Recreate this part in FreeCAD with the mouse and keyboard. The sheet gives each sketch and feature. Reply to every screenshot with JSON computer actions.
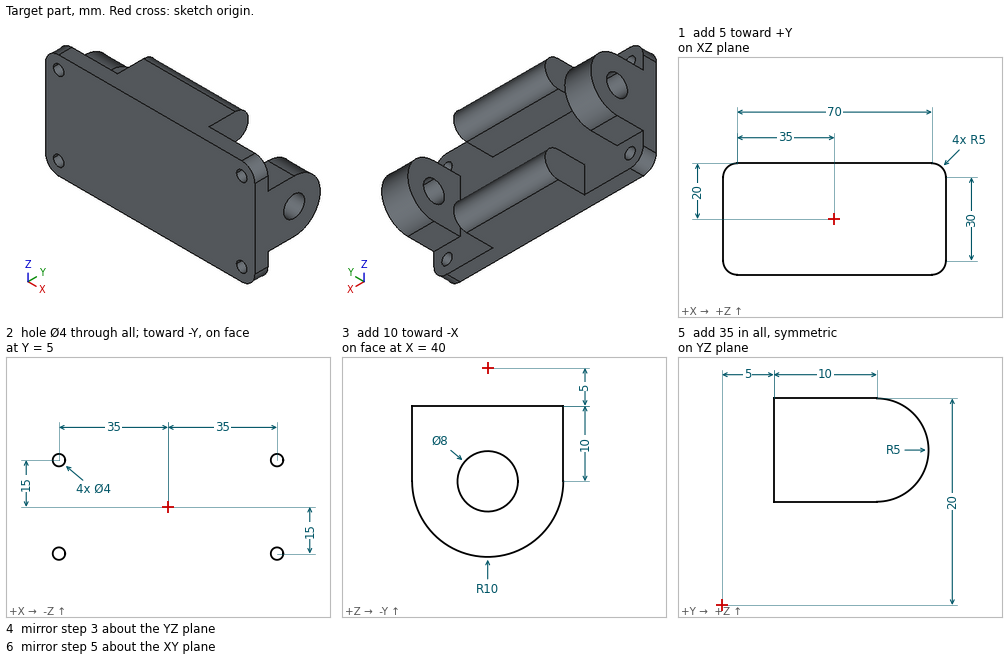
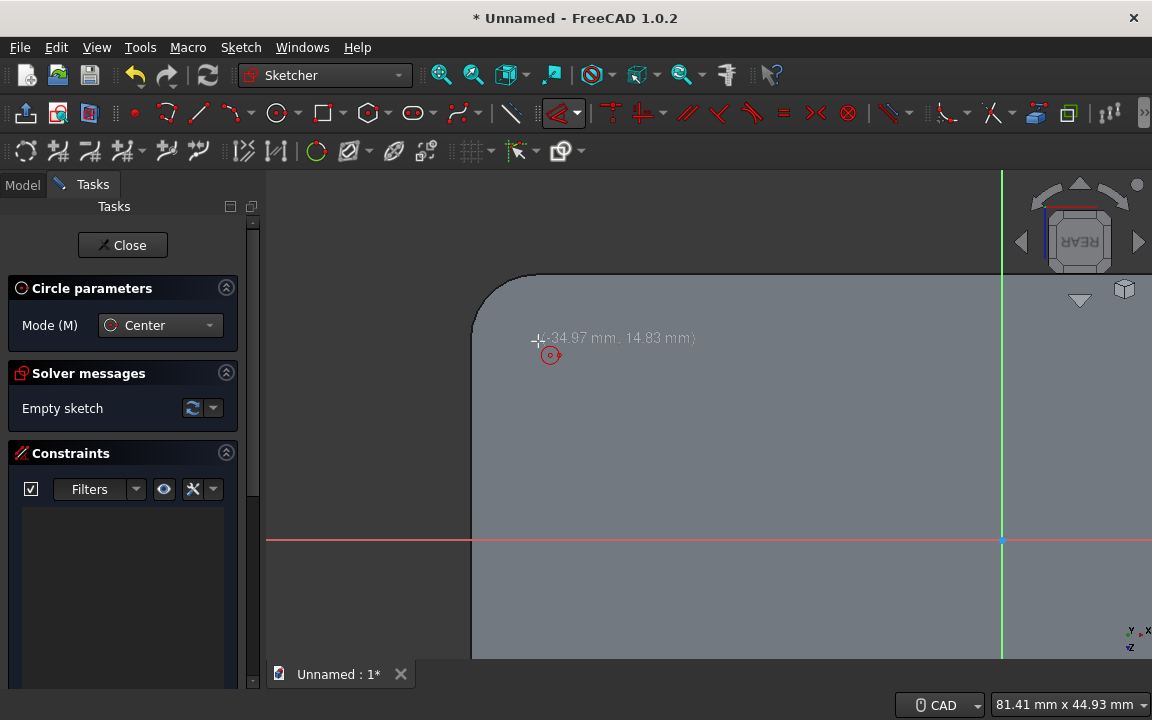
{"action": "left_click", "coordinate": [537, 341]}
{"action": "left_click", "coordinate": [556, 322]}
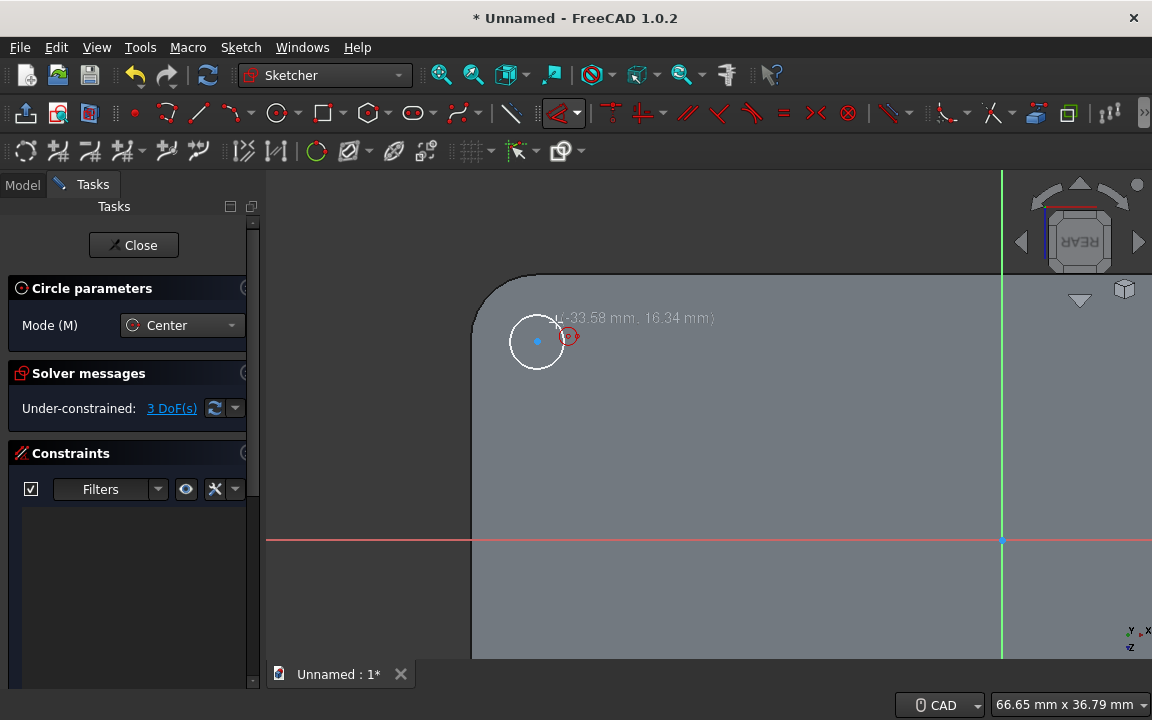
{"action": "scroll", "coordinate": [294, 262], "scroll_direction": "down", "scroll_amount": 3}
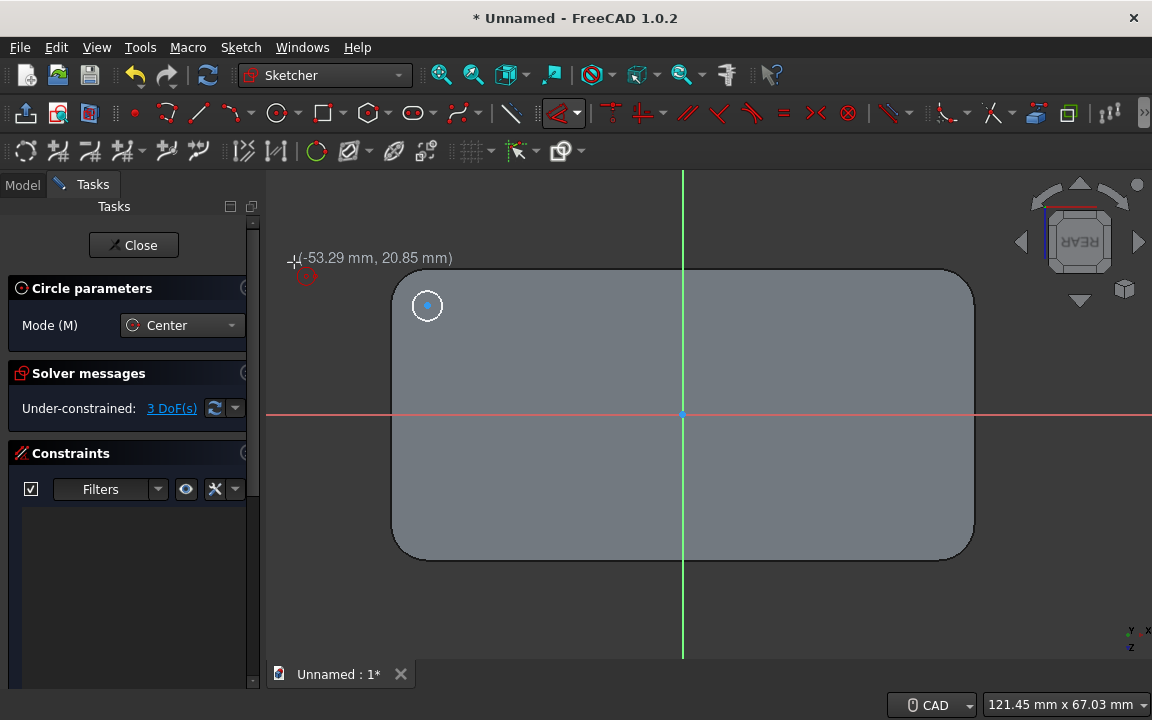
{"action": "scroll", "coordinate": [938, 305], "scroll_direction": "up", "scroll_amount": 3}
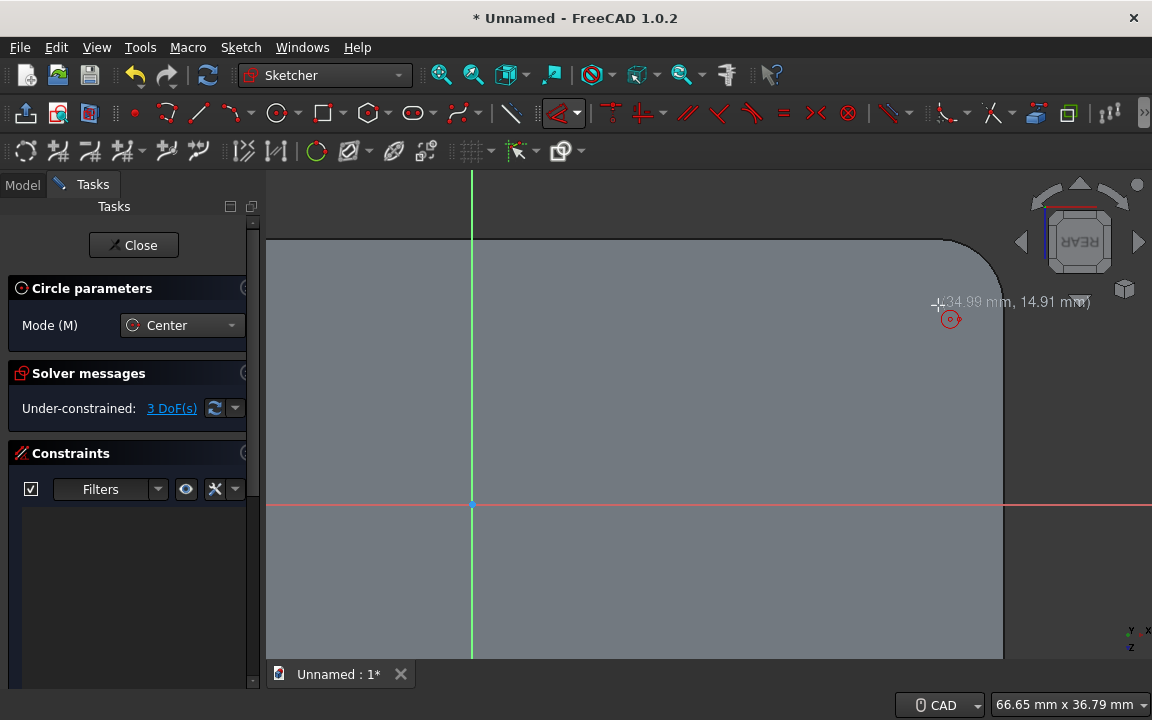
{"action": "left_click", "coordinate": [937, 305]}
{"action": "left_click", "coordinate": [956, 287]}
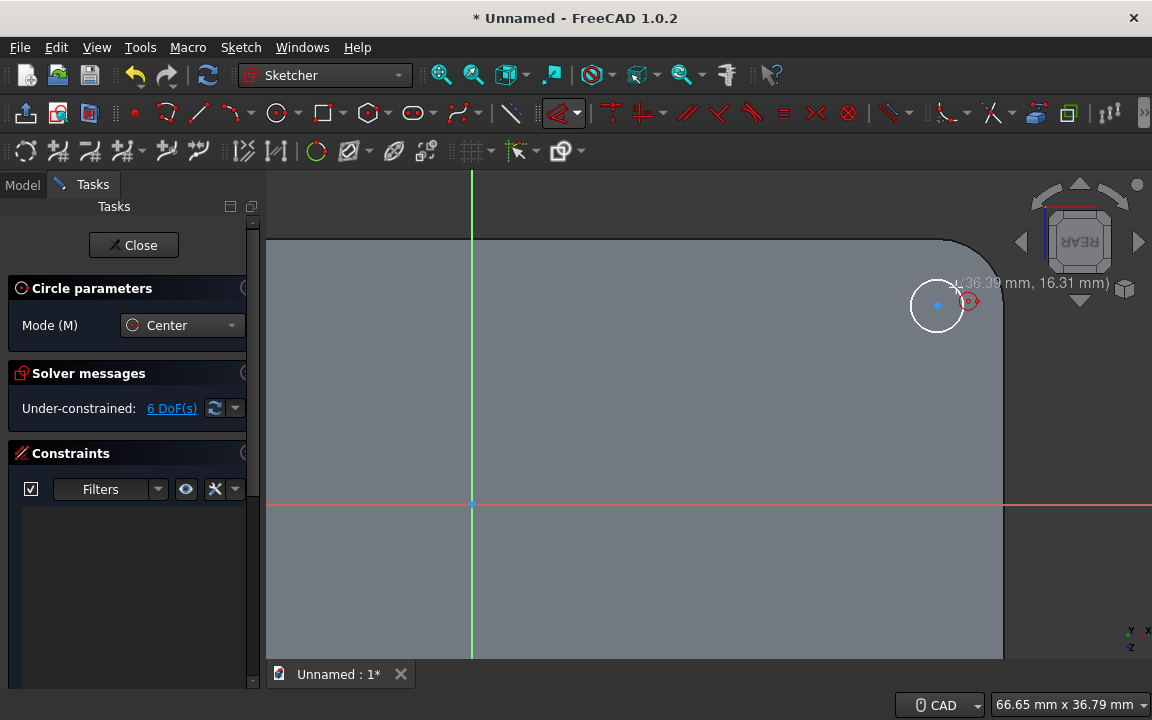
{"action": "scroll", "coordinate": [845, 305], "scroll_direction": "down", "scroll_amount": 3}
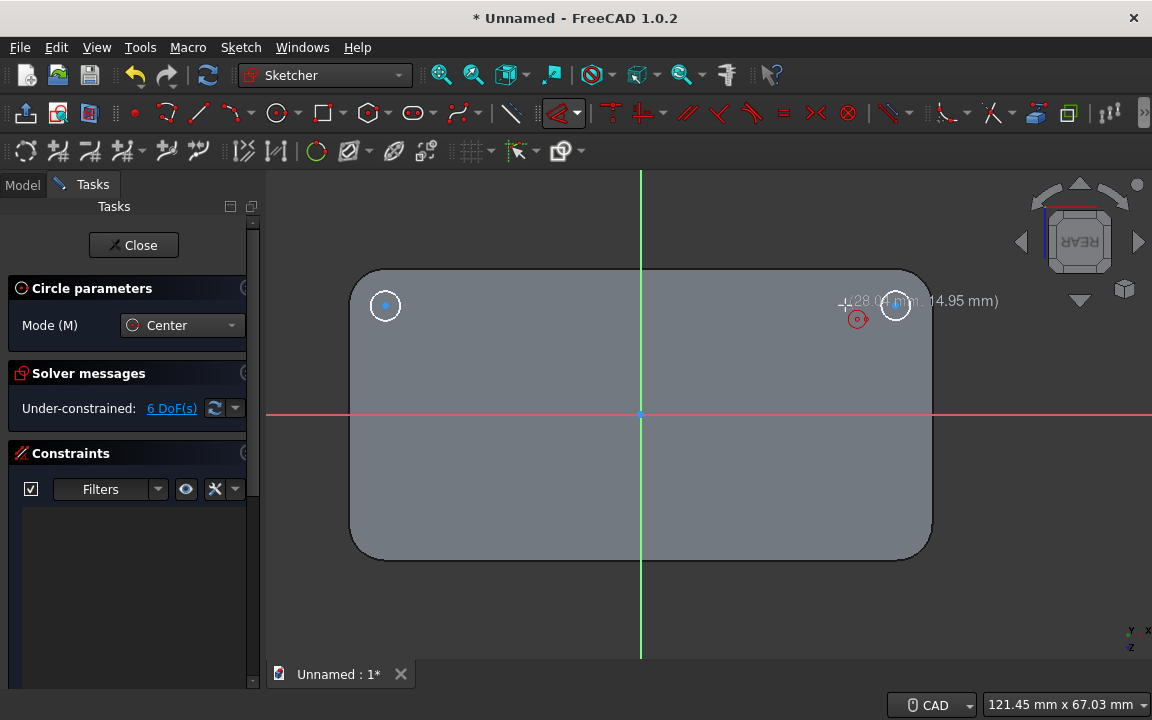
{"action": "scroll", "coordinate": [896, 524], "scroll_direction": "up", "scroll_amount": 3}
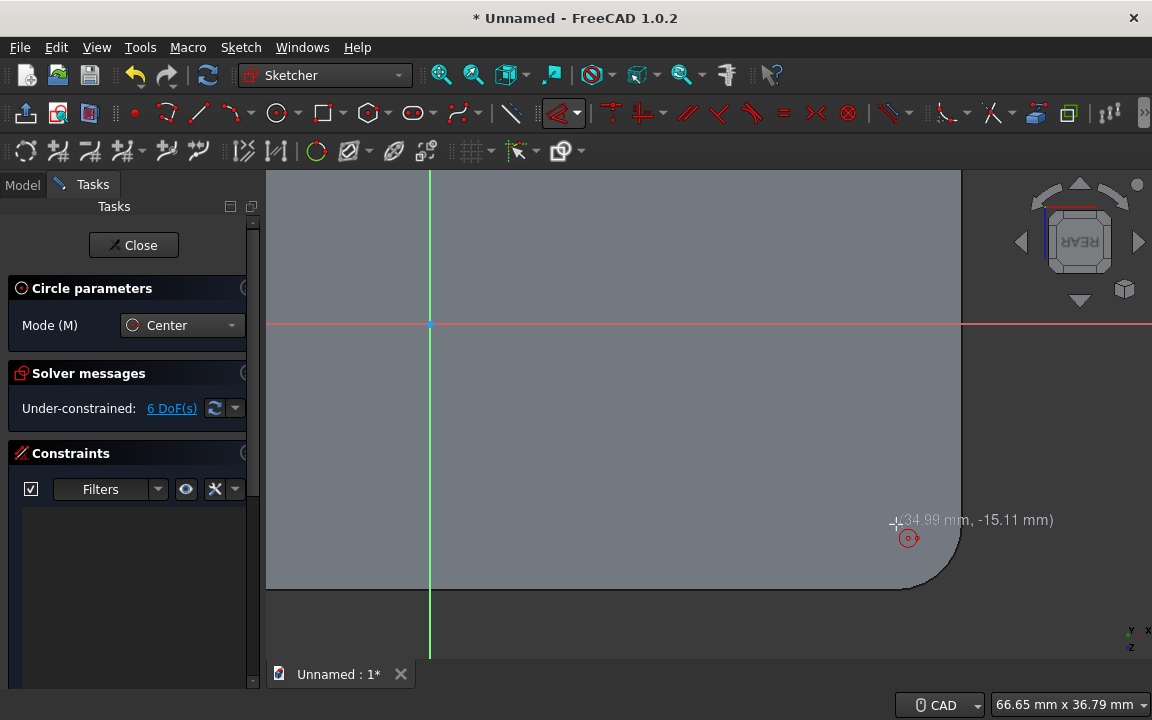
{"action": "left_click", "coordinate": [896, 524]}
{"action": "left_click", "coordinate": [914, 505]}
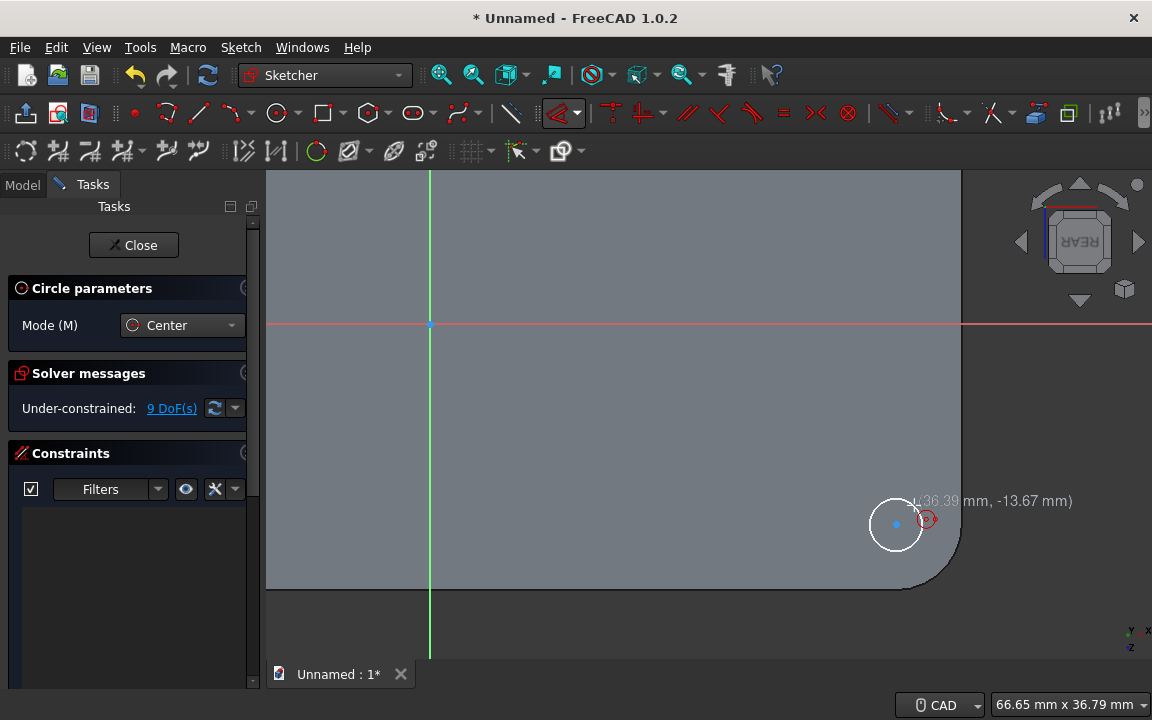
{"action": "scroll", "coordinate": [896, 524], "scroll_direction": "down", "scroll_amount": 3}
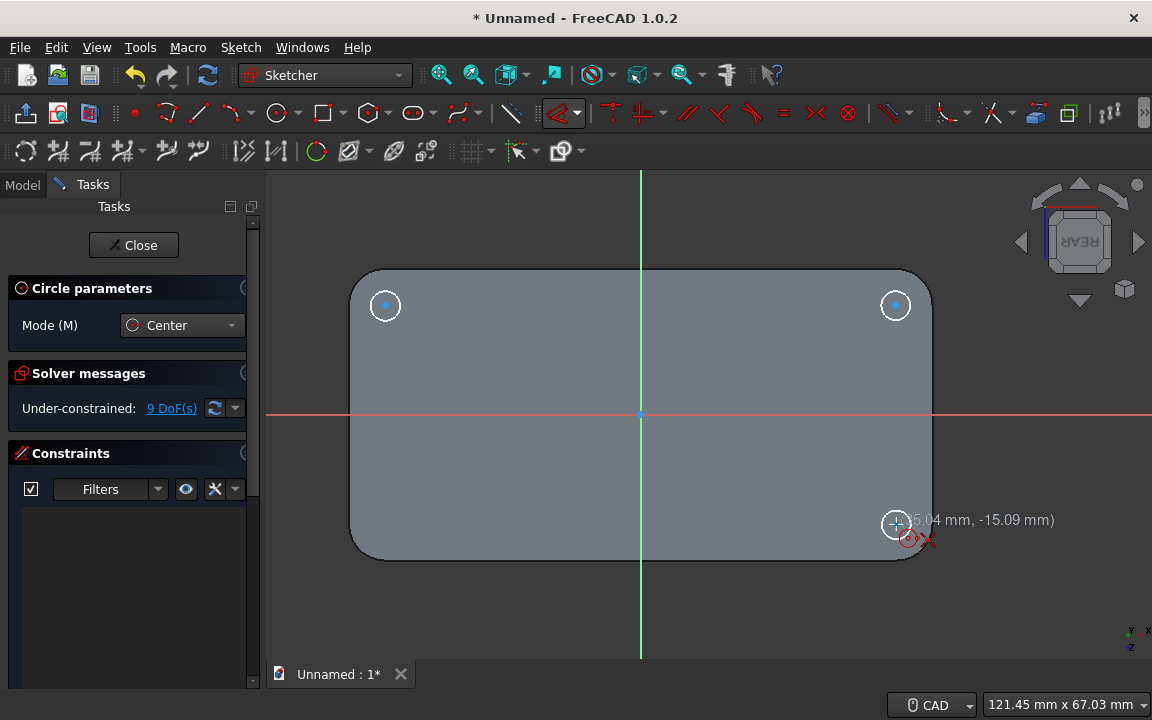
{"action": "scroll", "coordinate": [385, 524], "scroll_direction": "up", "scroll_amount": 3}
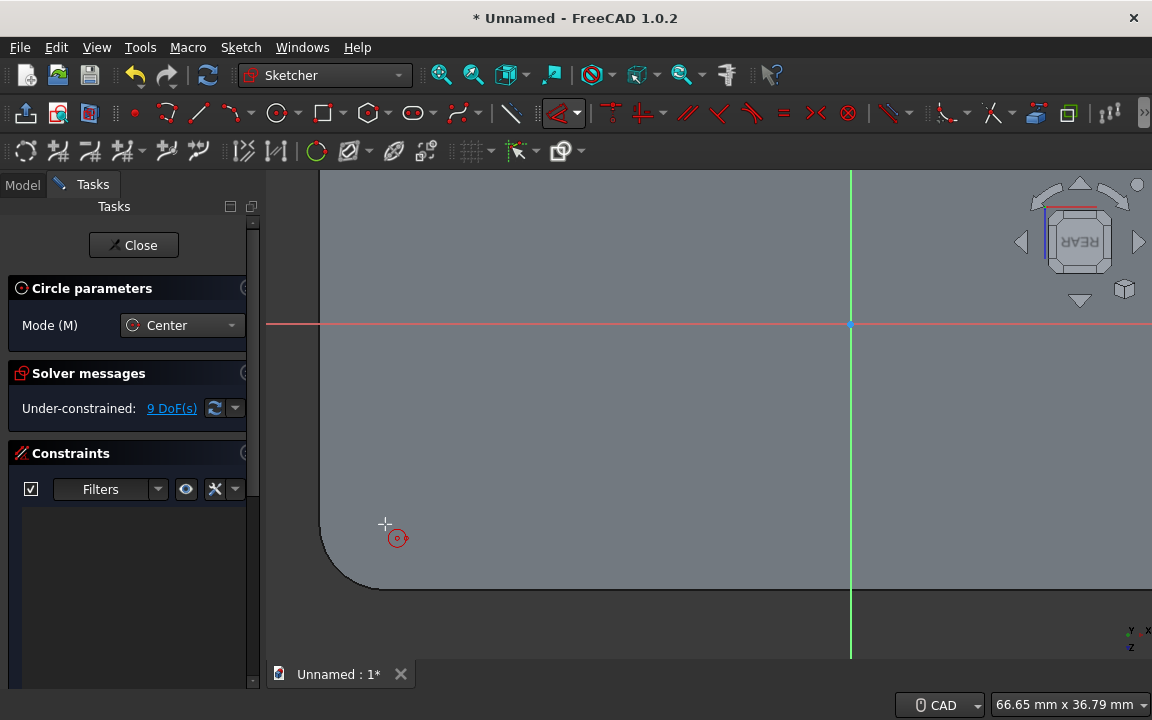
{"action": "left_click", "coordinate": [386, 524]}
{"action": "left_click", "coordinate": [404, 505]}
{"action": "key", "text": "Escape"}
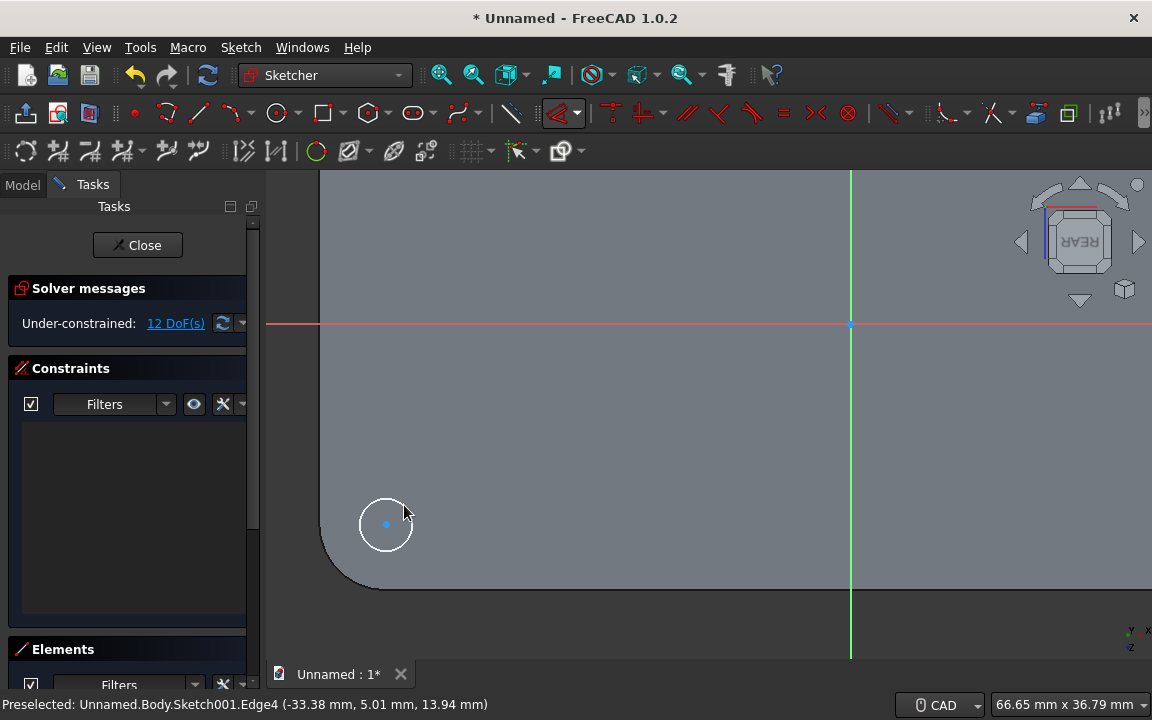
{"action": "scroll", "coordinate": [385, 524], "scroll_direction": "down", "scroll_amount": 3}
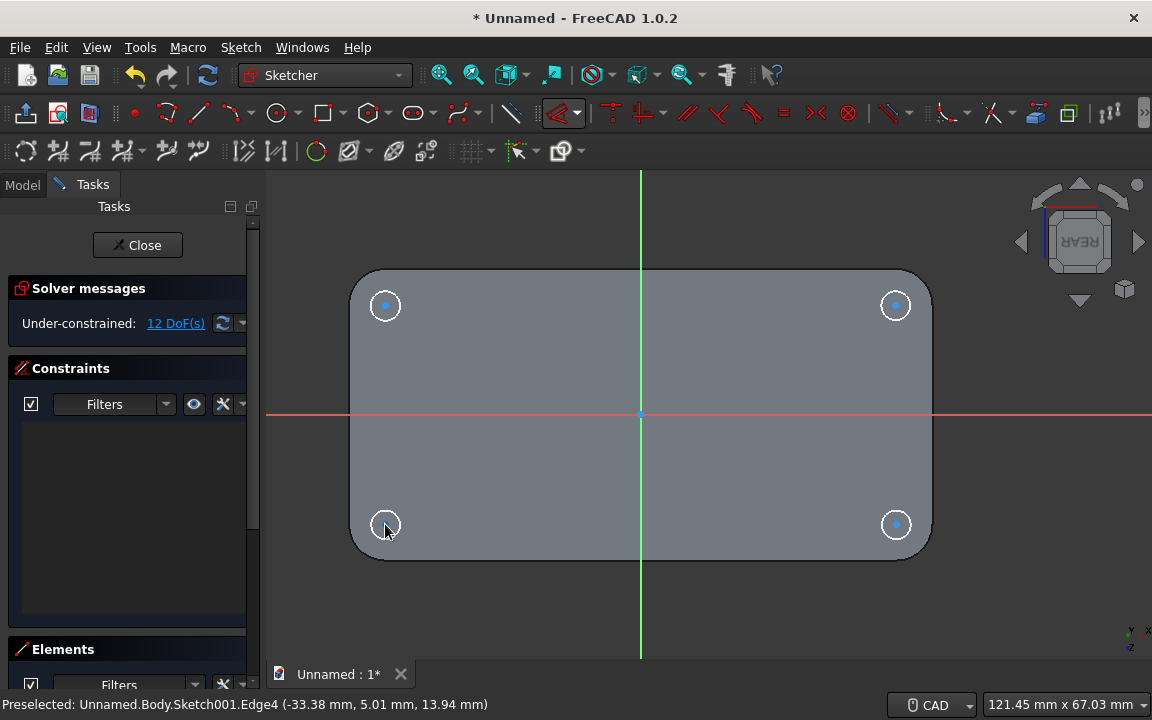
{"action": "left_click", "coordinate": [396, 296]}